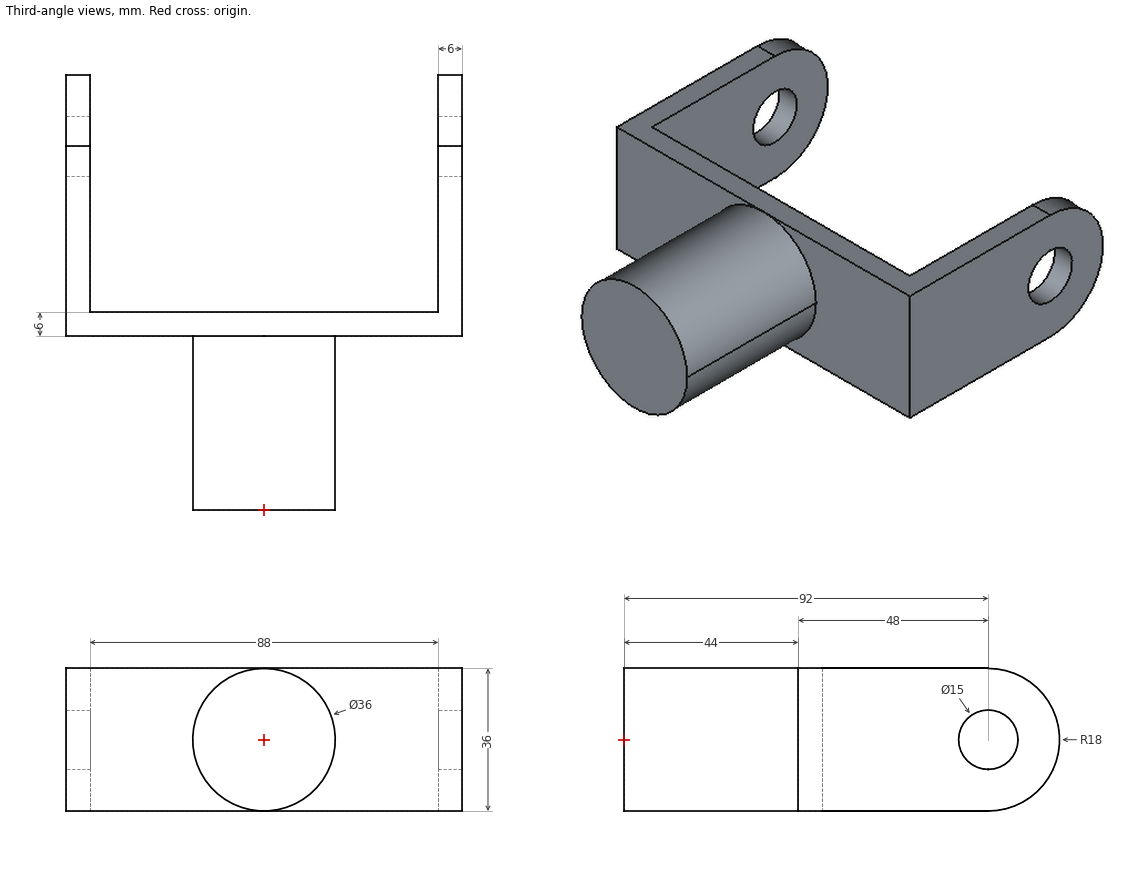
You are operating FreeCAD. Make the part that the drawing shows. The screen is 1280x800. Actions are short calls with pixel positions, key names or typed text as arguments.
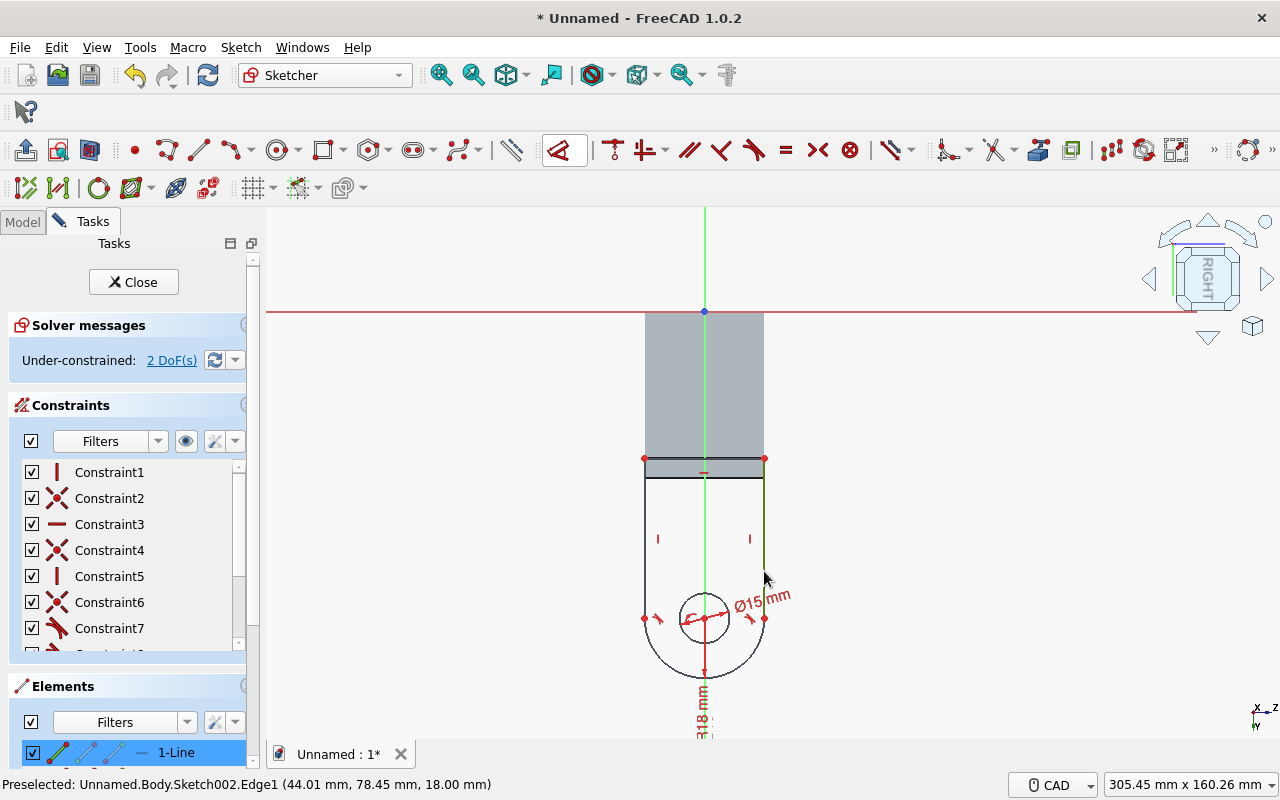
key(i)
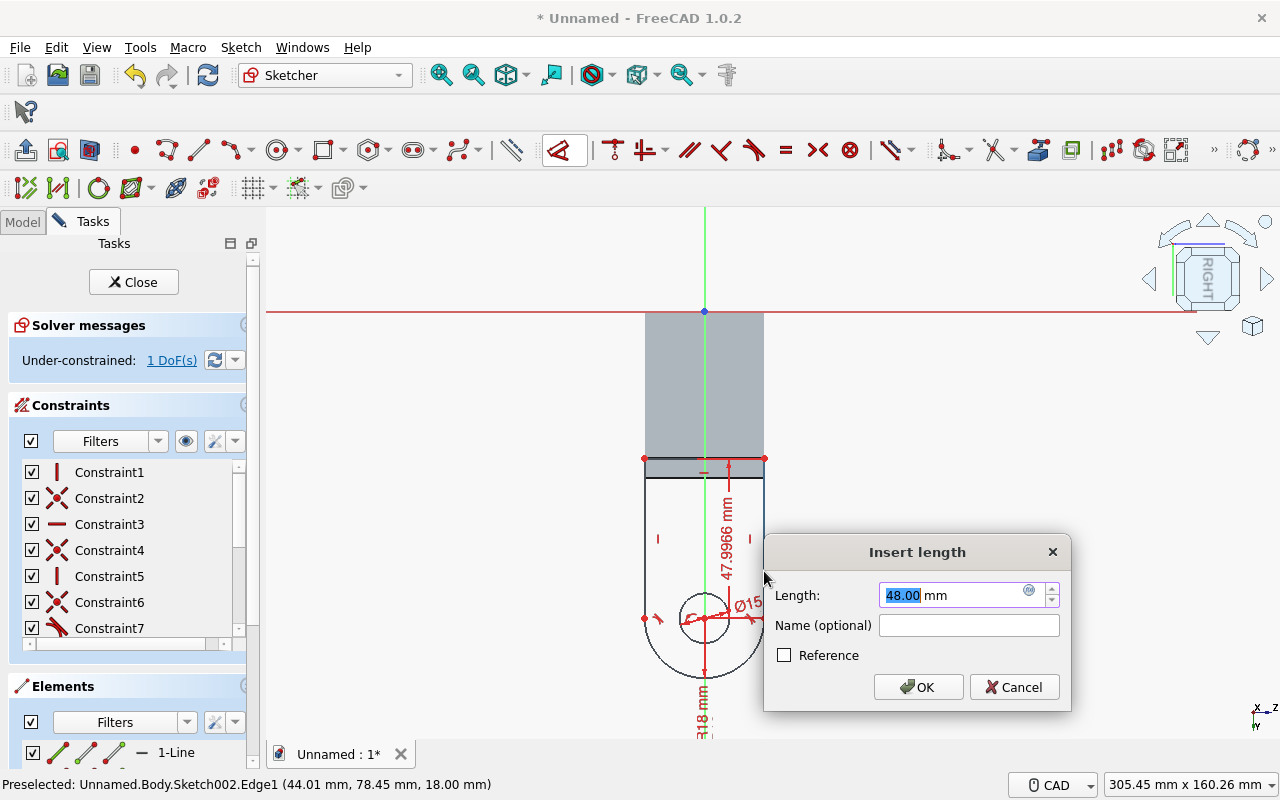
text(48)
key(Return)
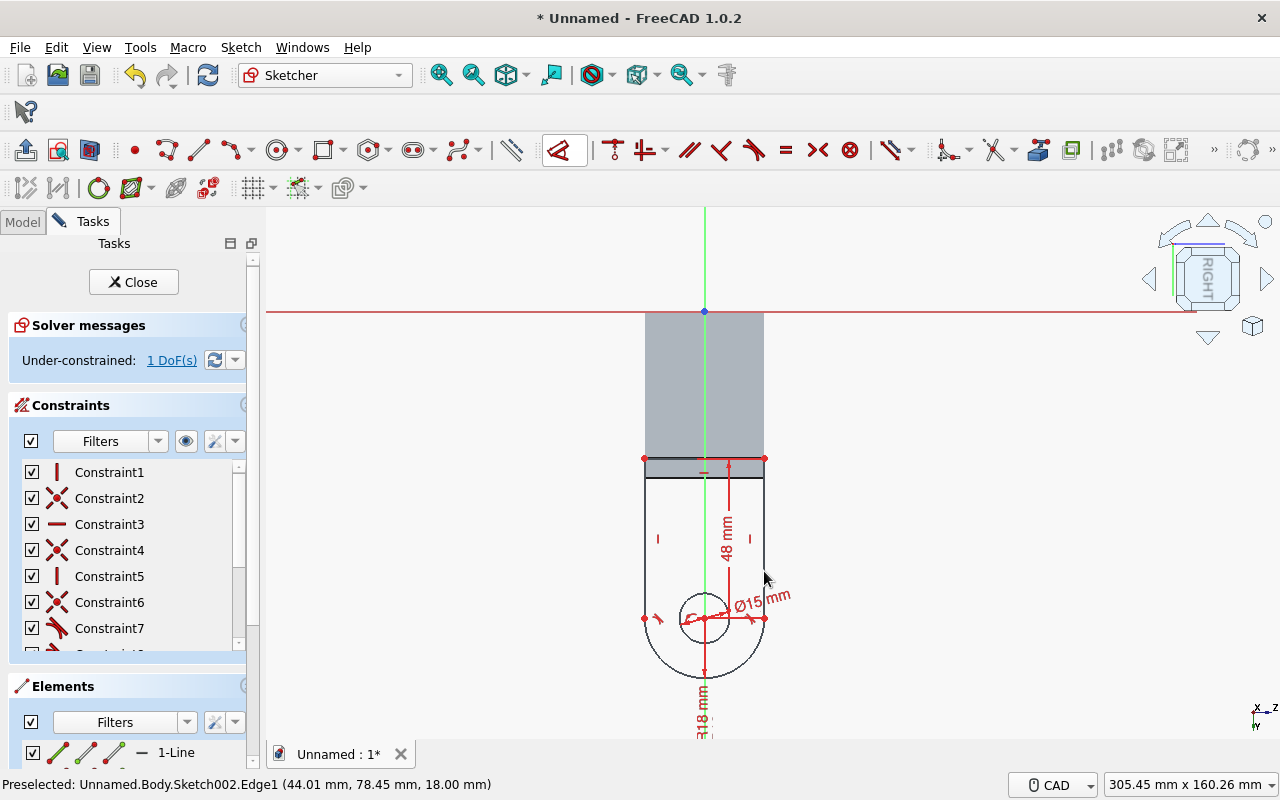
click(705, 618)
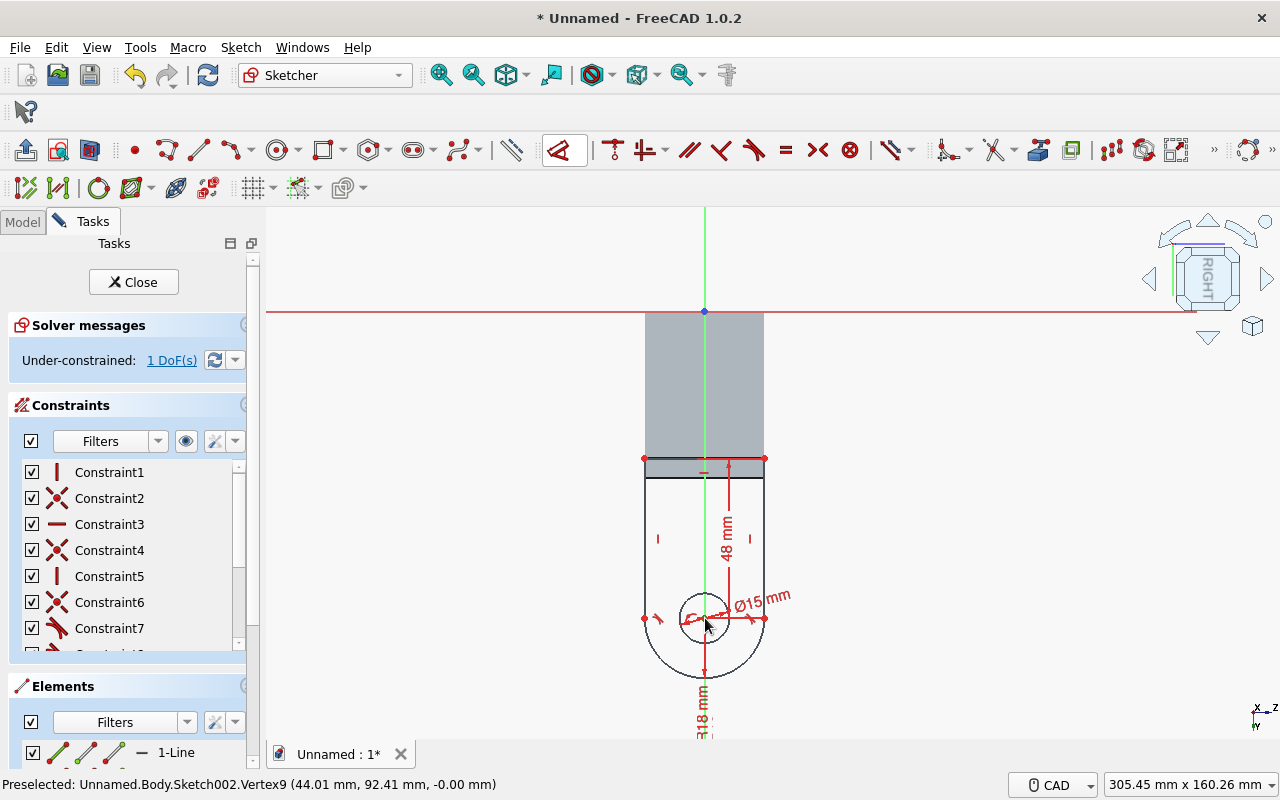
key(i)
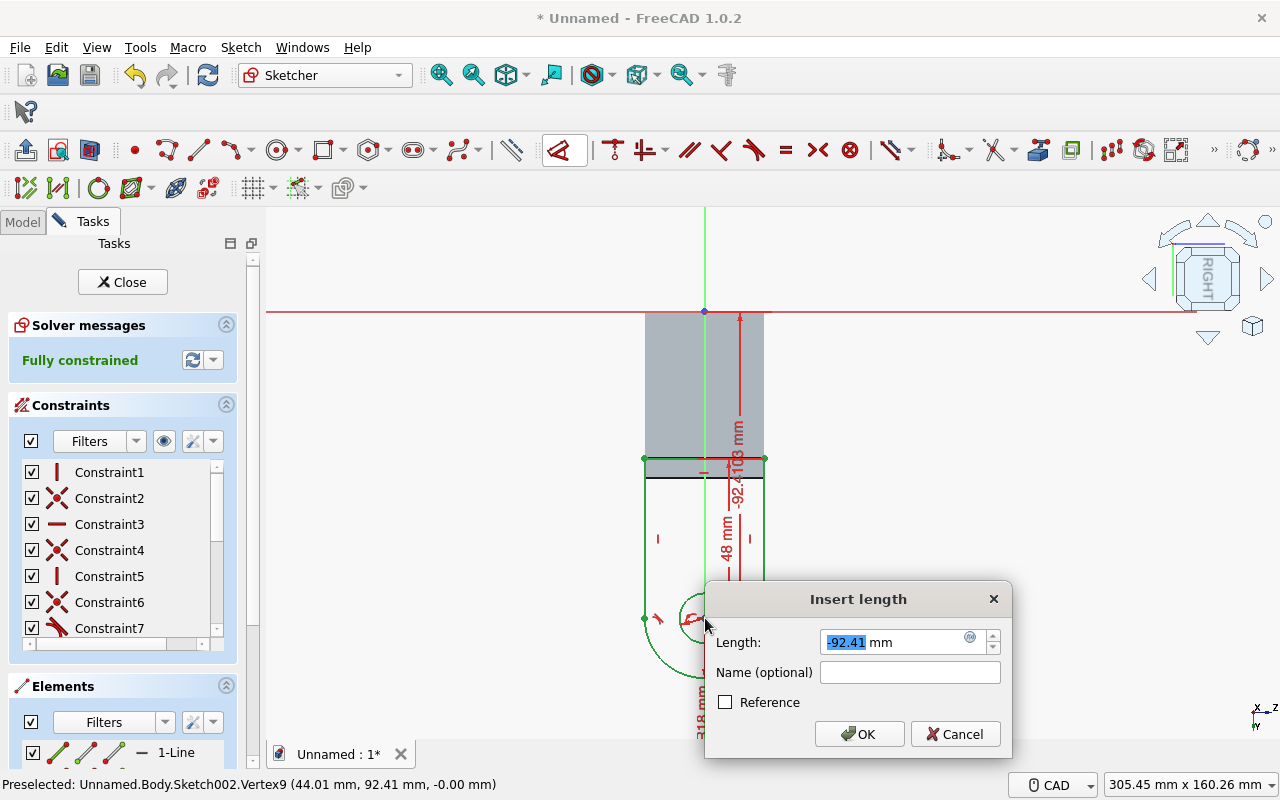
text(-92)
key(Return)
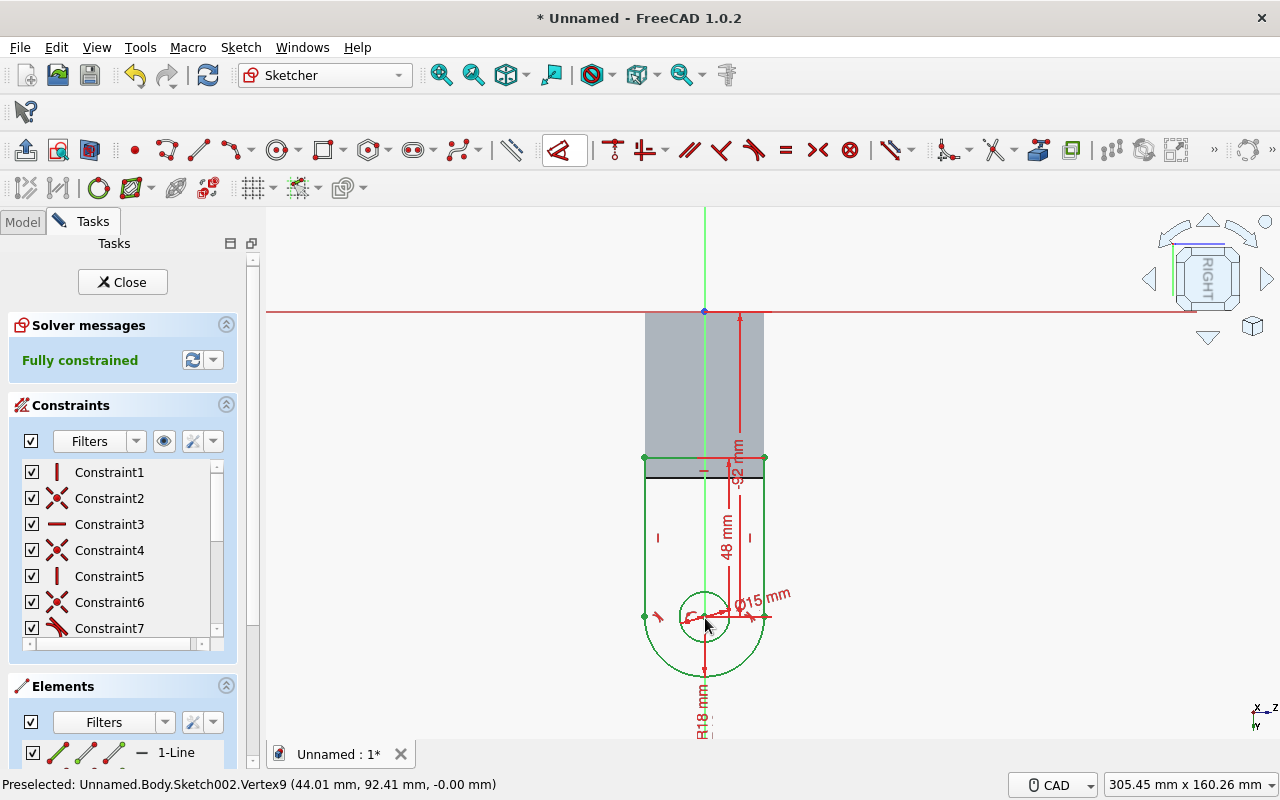
click(123, 282)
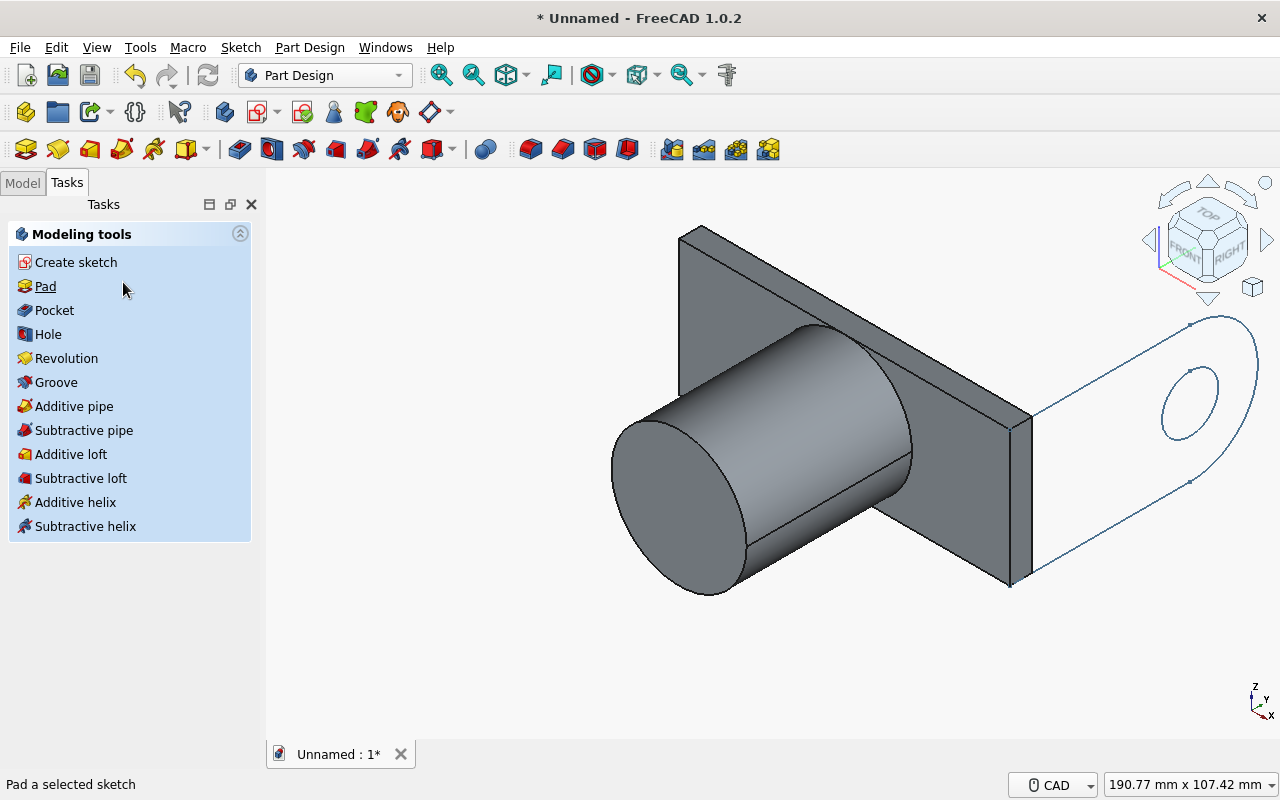
click(26, 150)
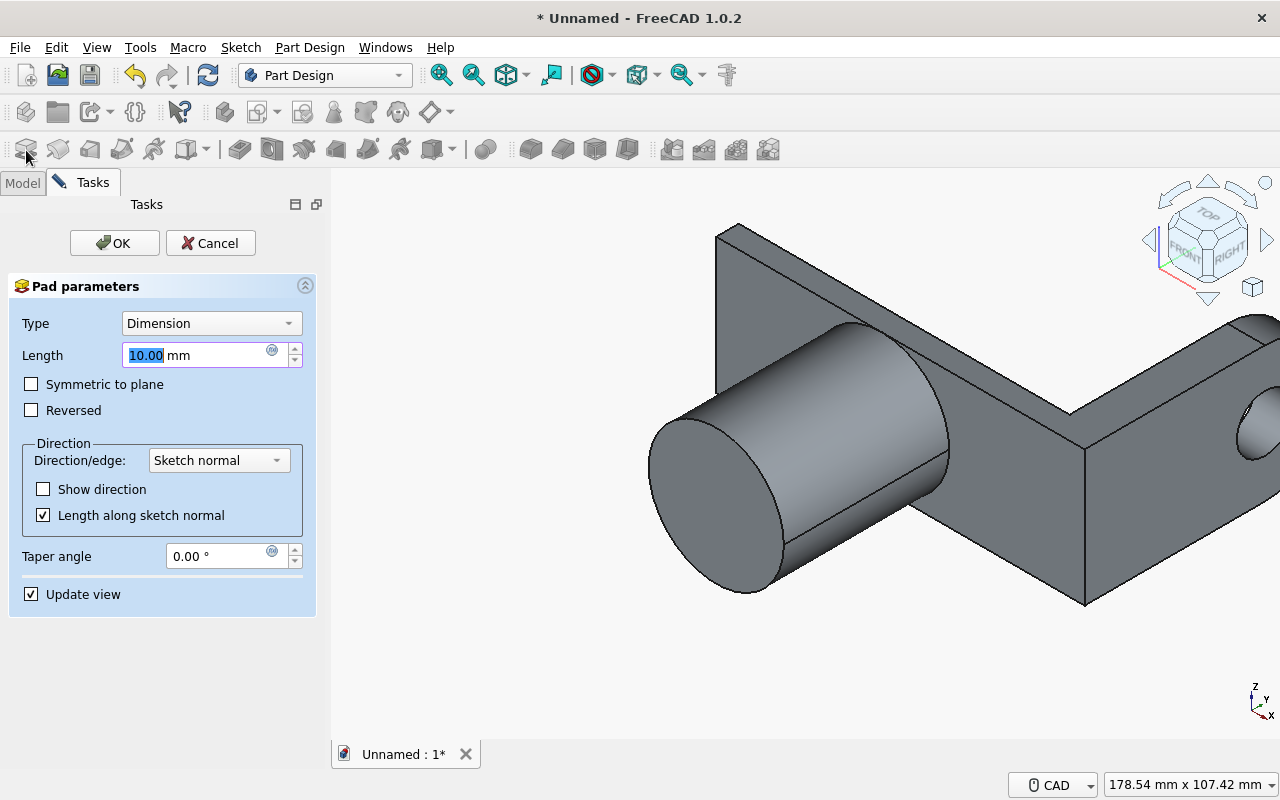
text(6)
key(Tab)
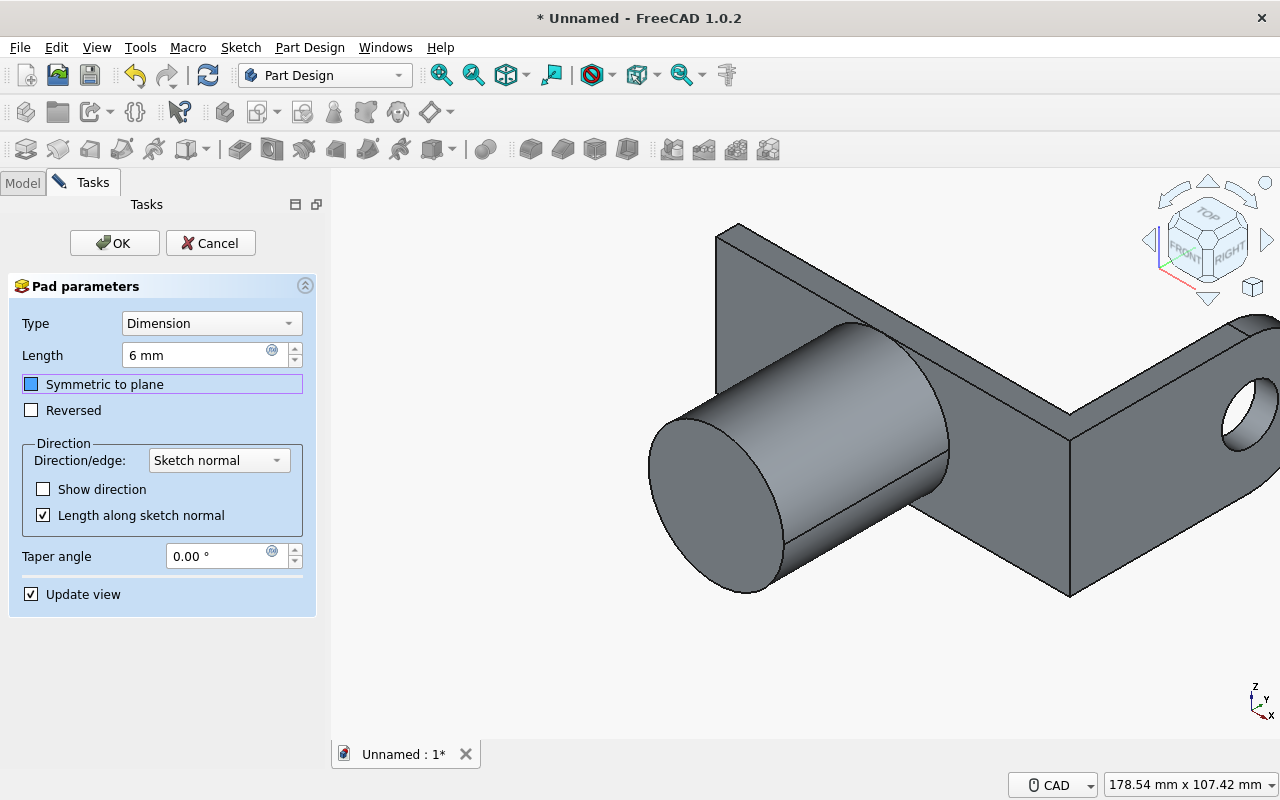
click(115, 243)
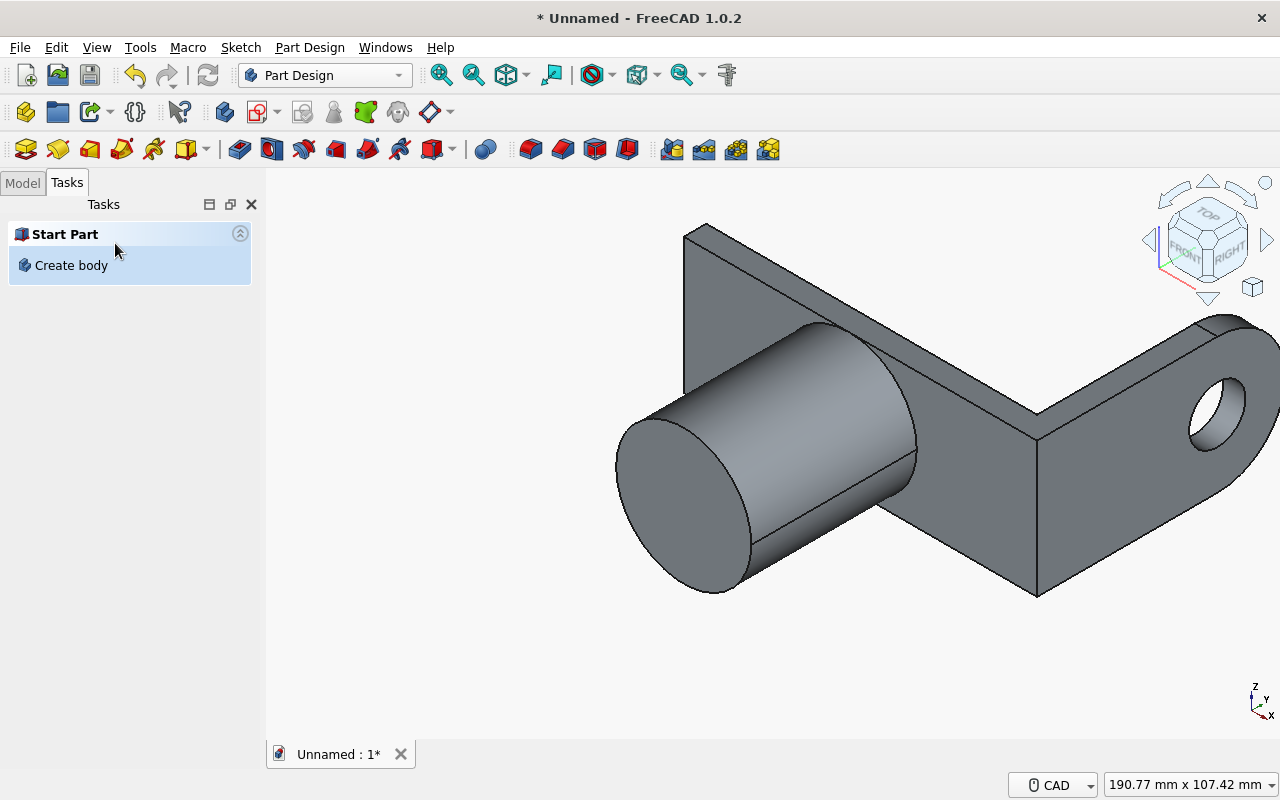
key(v)
key(f)